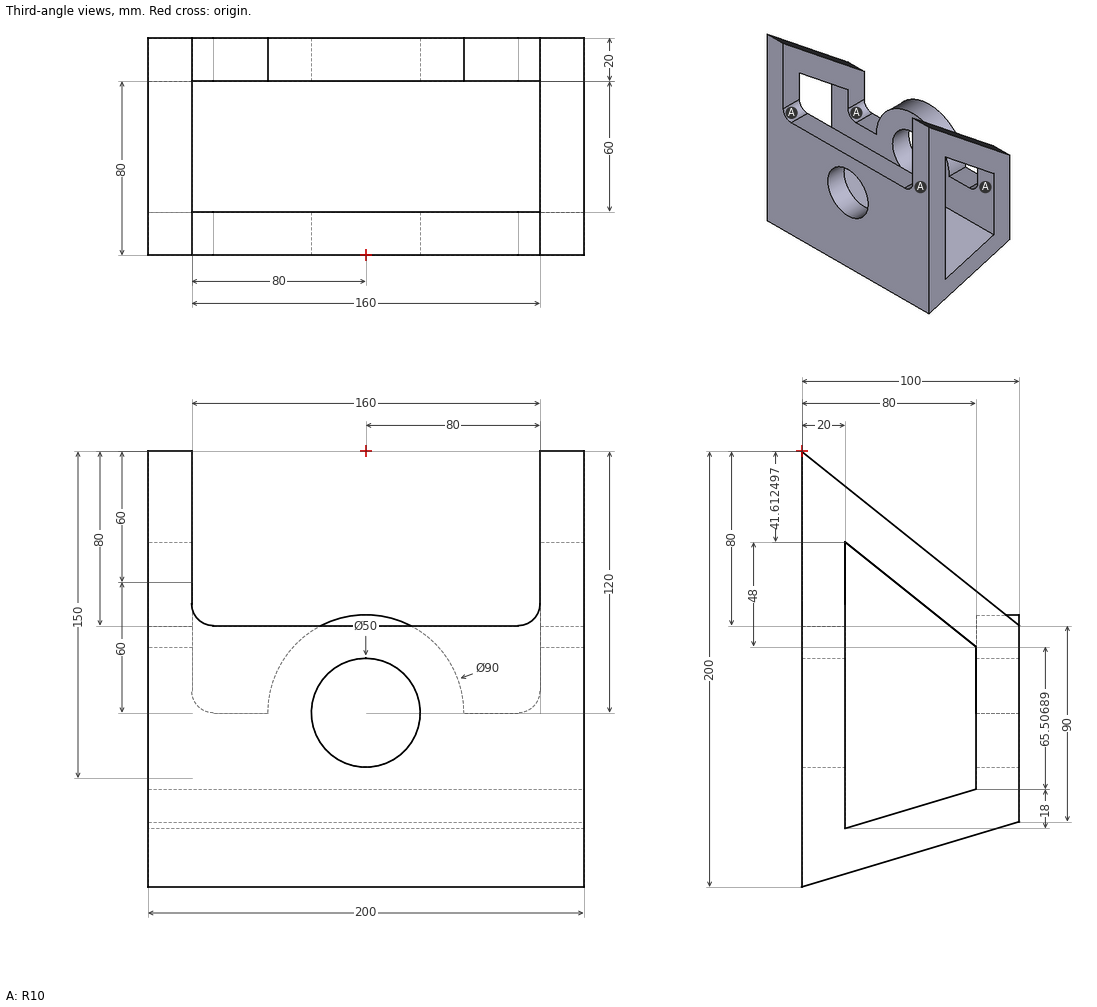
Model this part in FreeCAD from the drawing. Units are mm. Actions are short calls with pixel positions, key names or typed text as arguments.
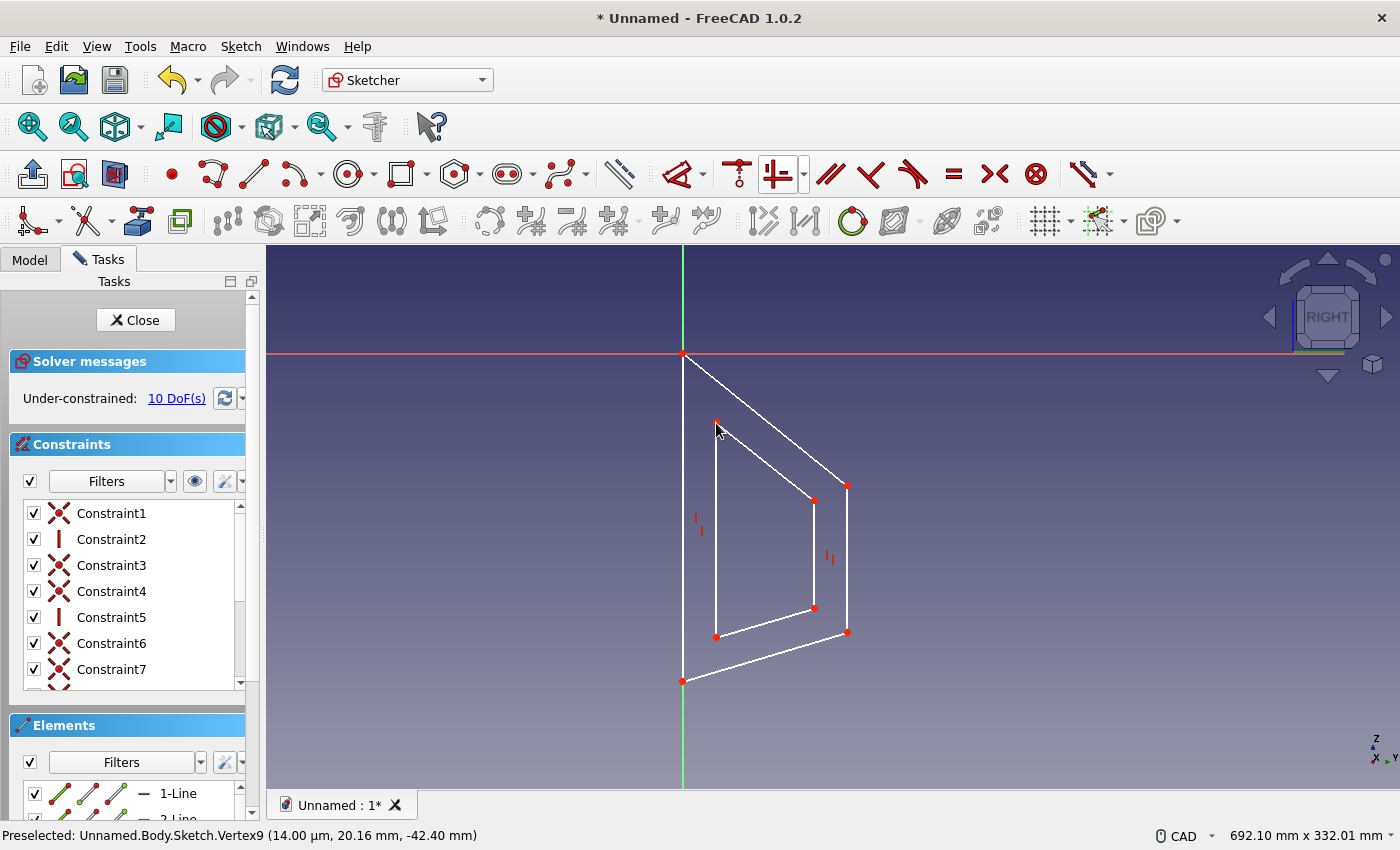
key(d)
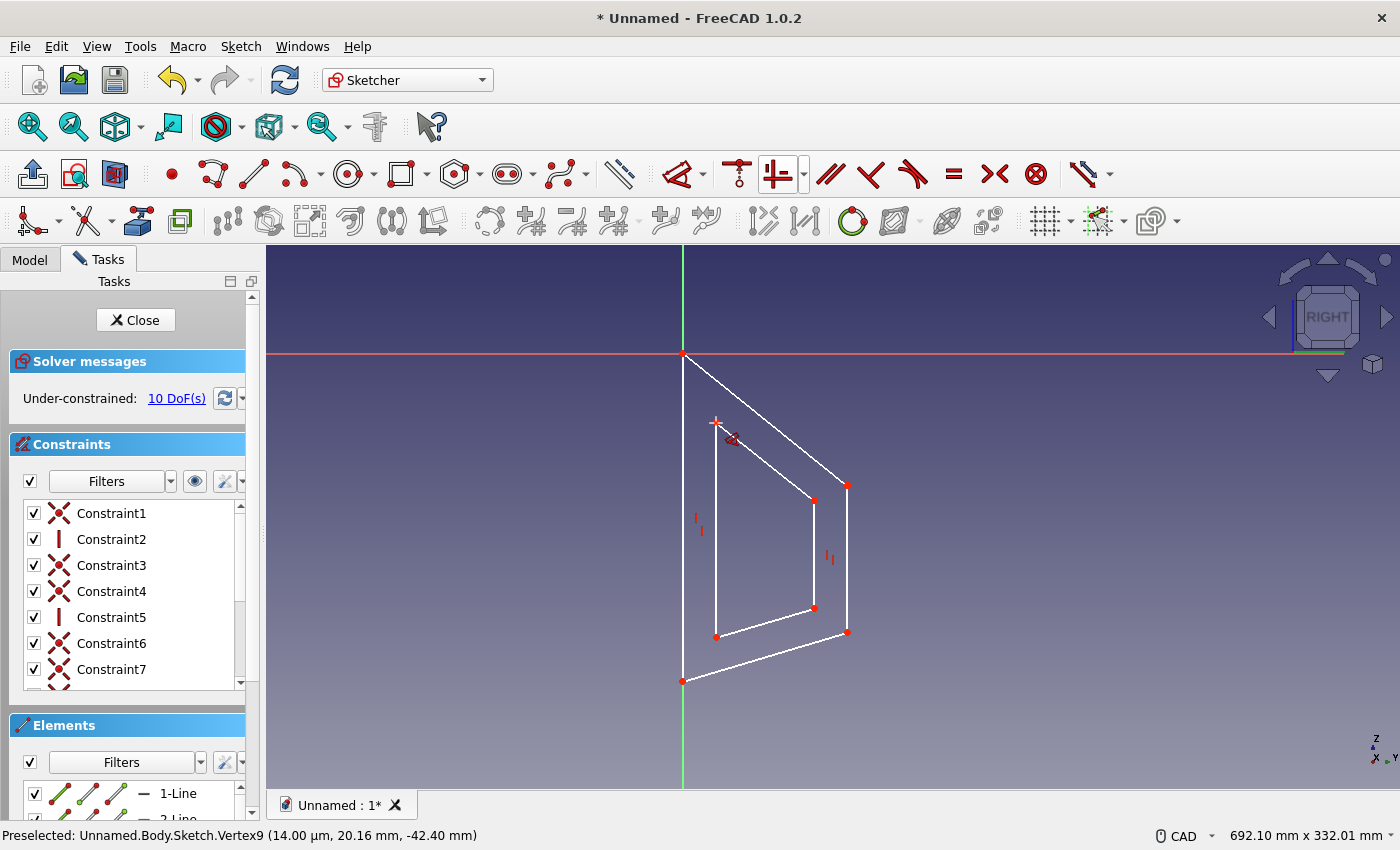
click(847, 589)
click(881, 559)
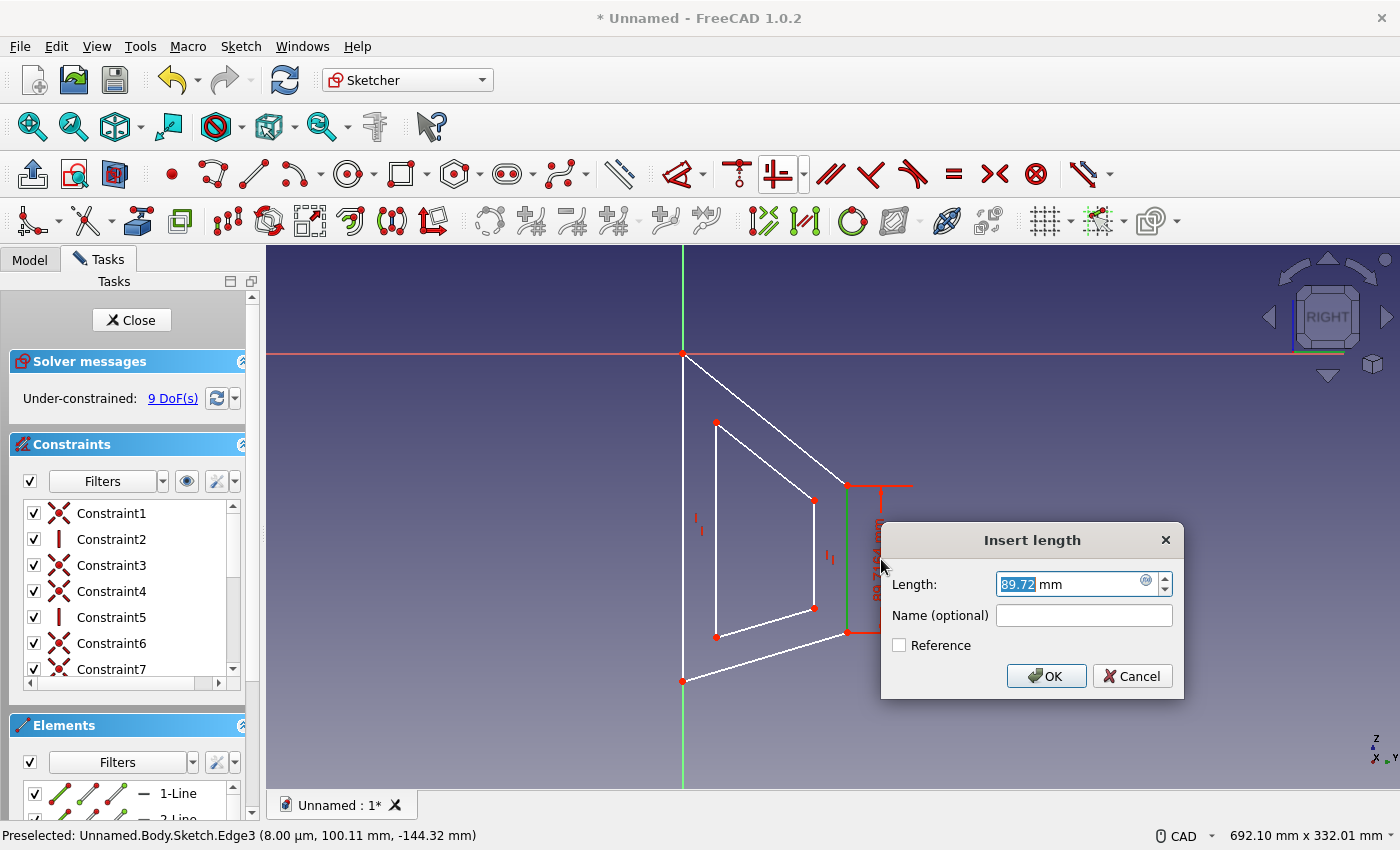
text(90)
key(Return)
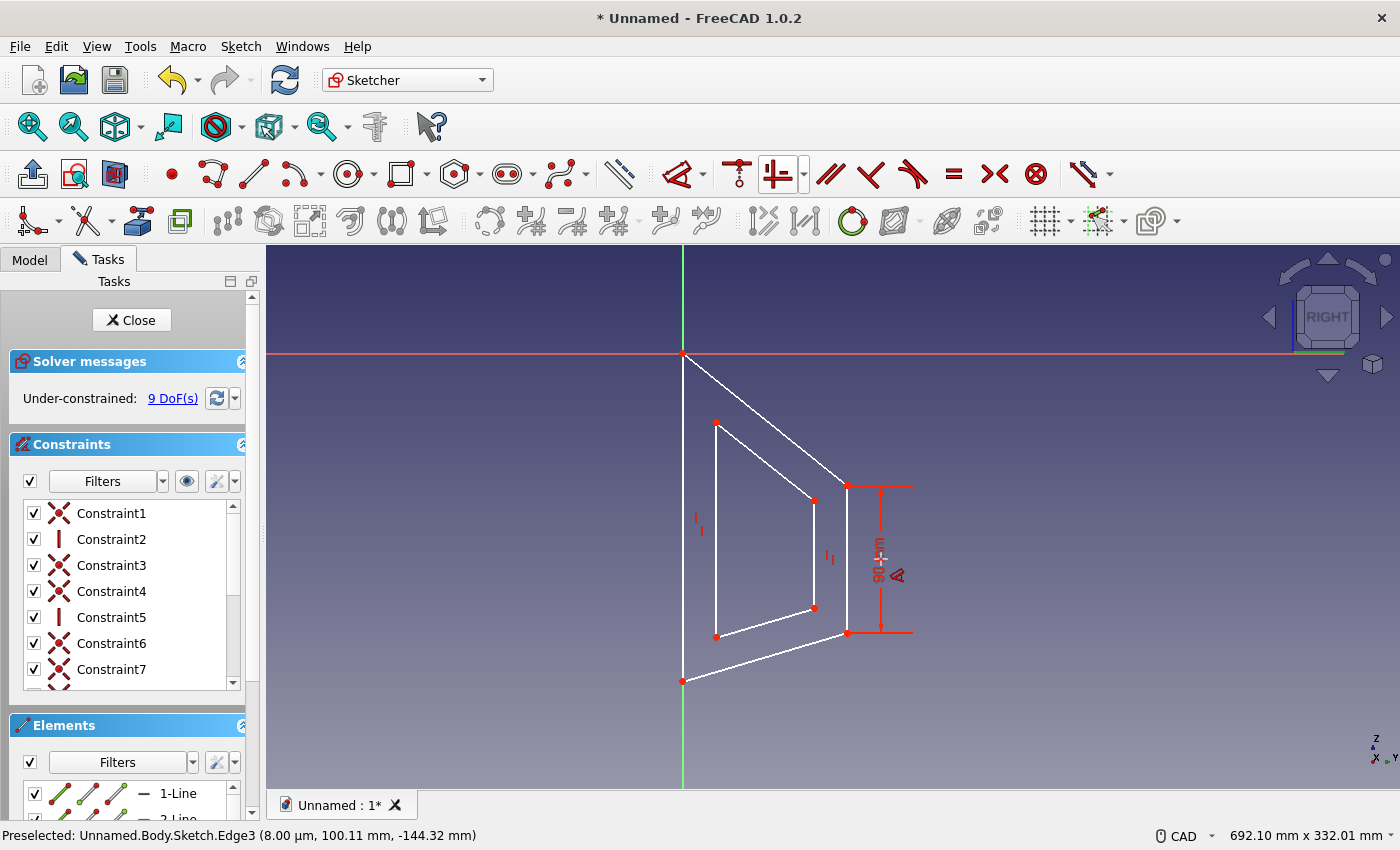
click(683, 452)
click(649, 518)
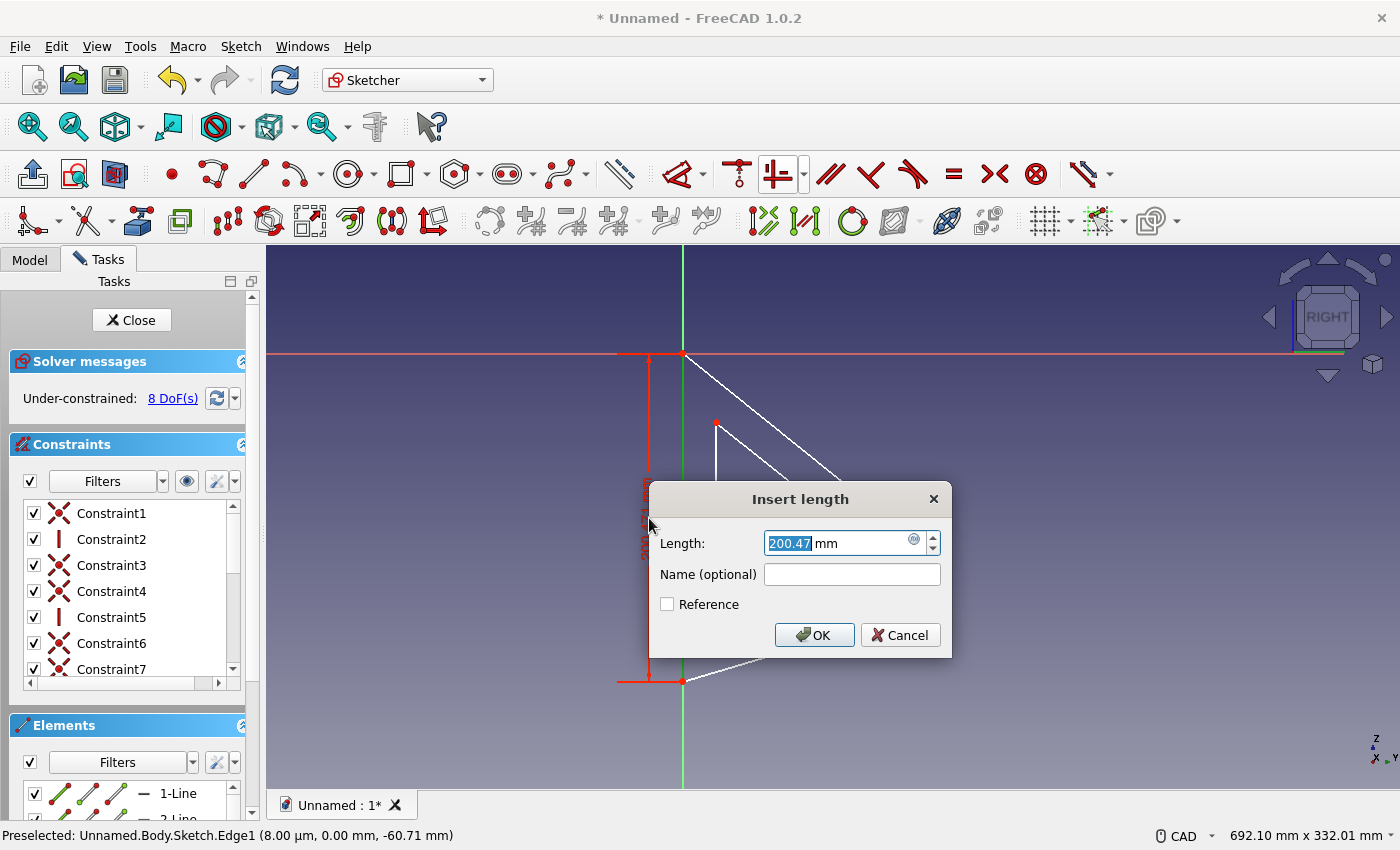
text(200)
key(Return)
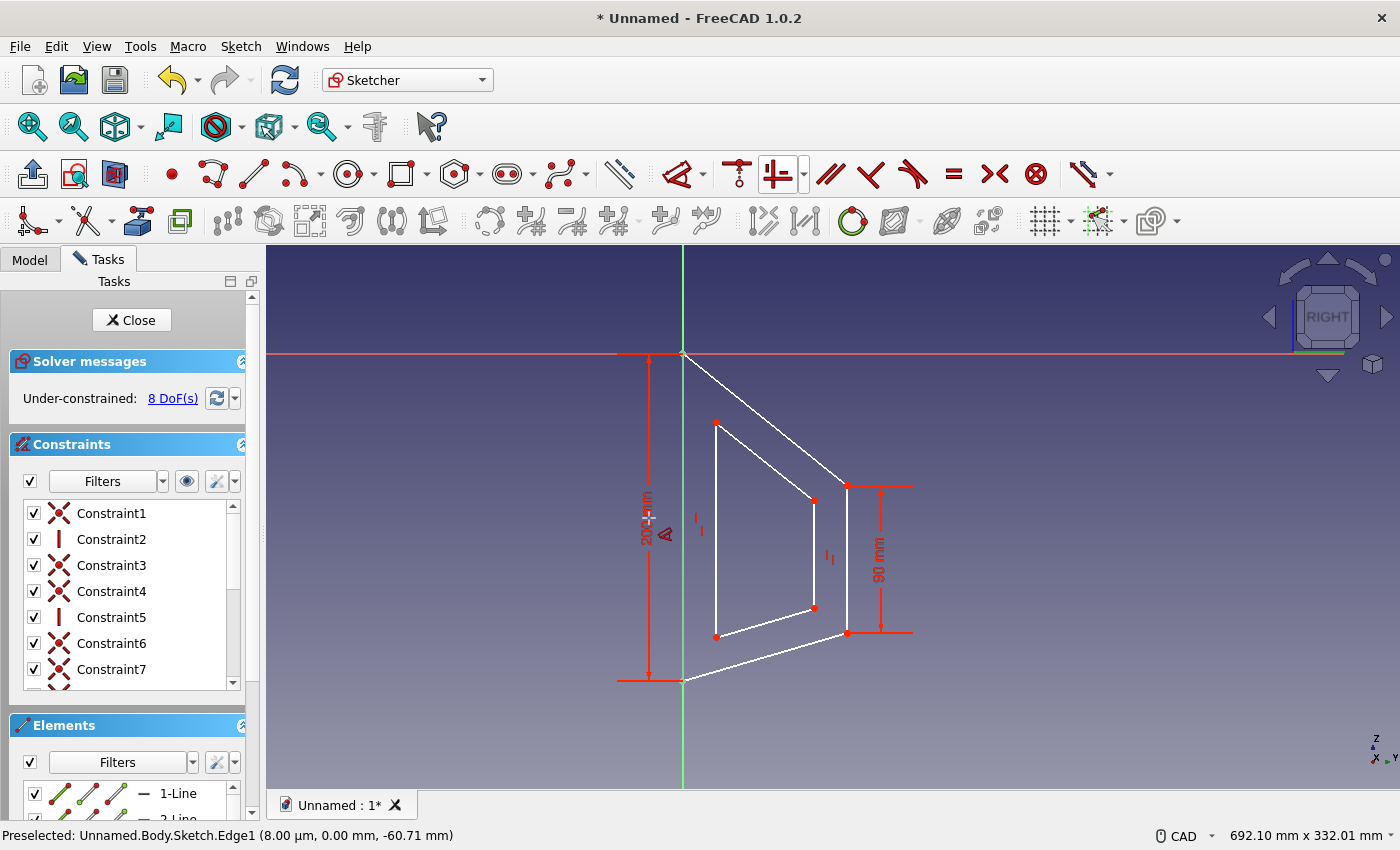
click(847, 486)
click(881, 420)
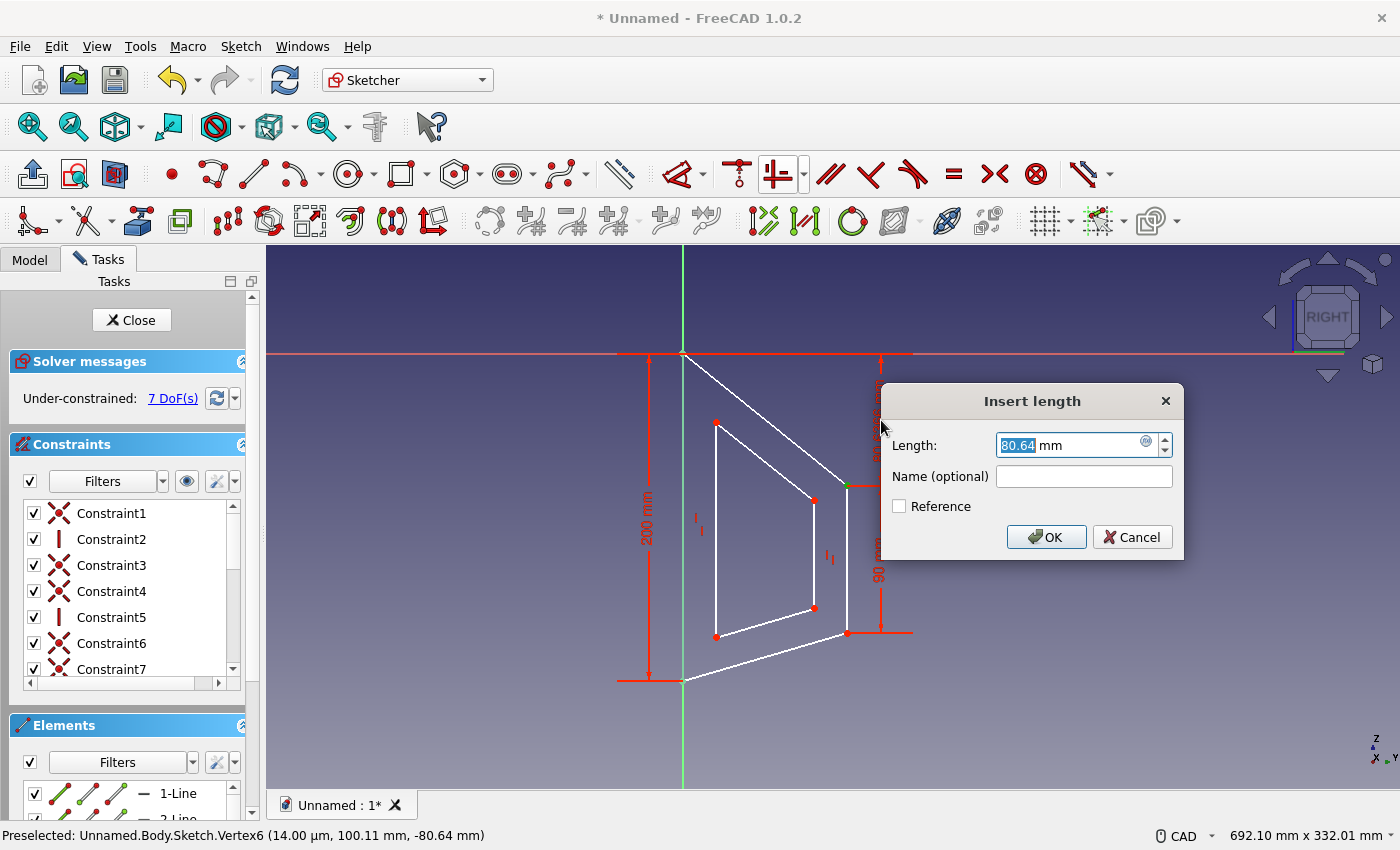
text(80)
key(Return)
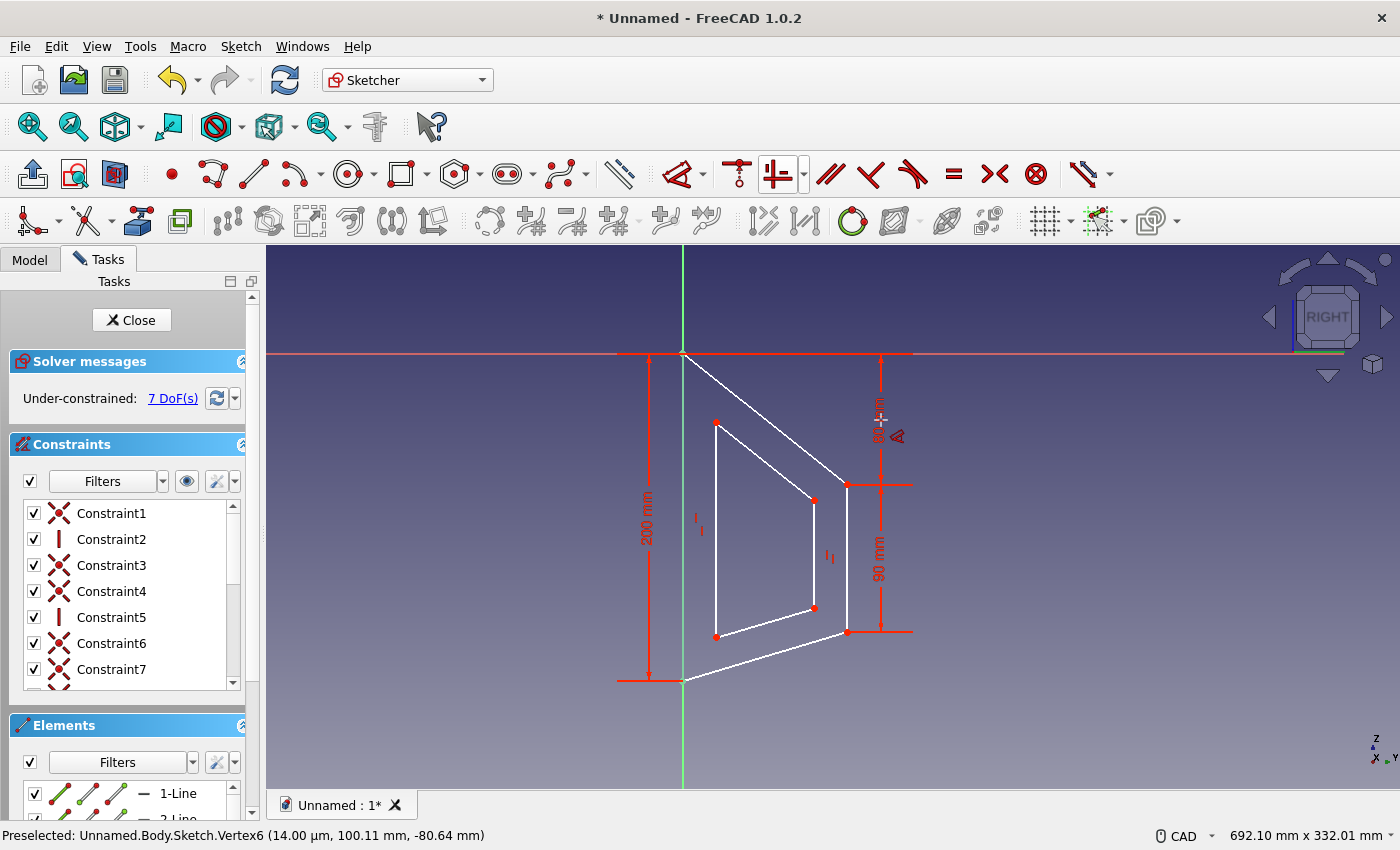
click(716, 423)
click(699, 320)